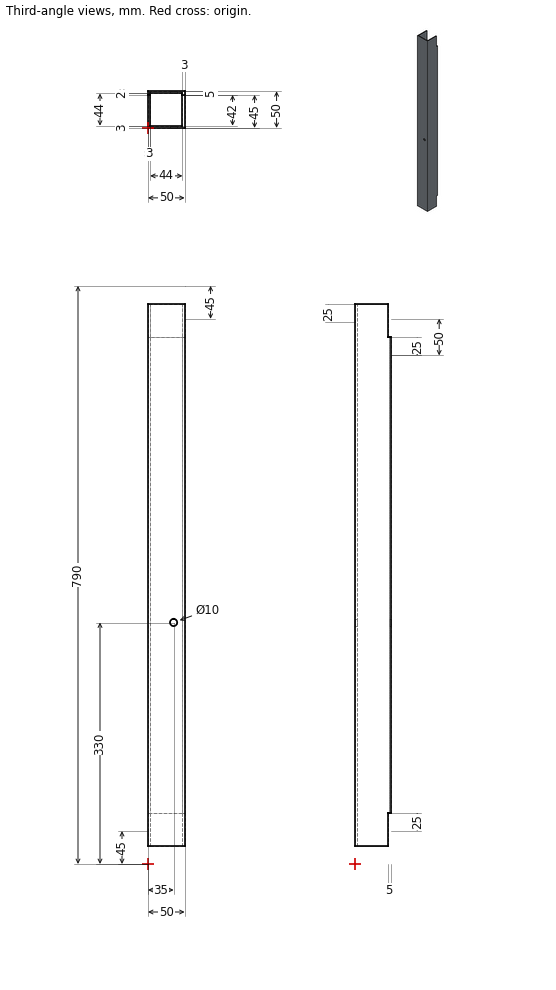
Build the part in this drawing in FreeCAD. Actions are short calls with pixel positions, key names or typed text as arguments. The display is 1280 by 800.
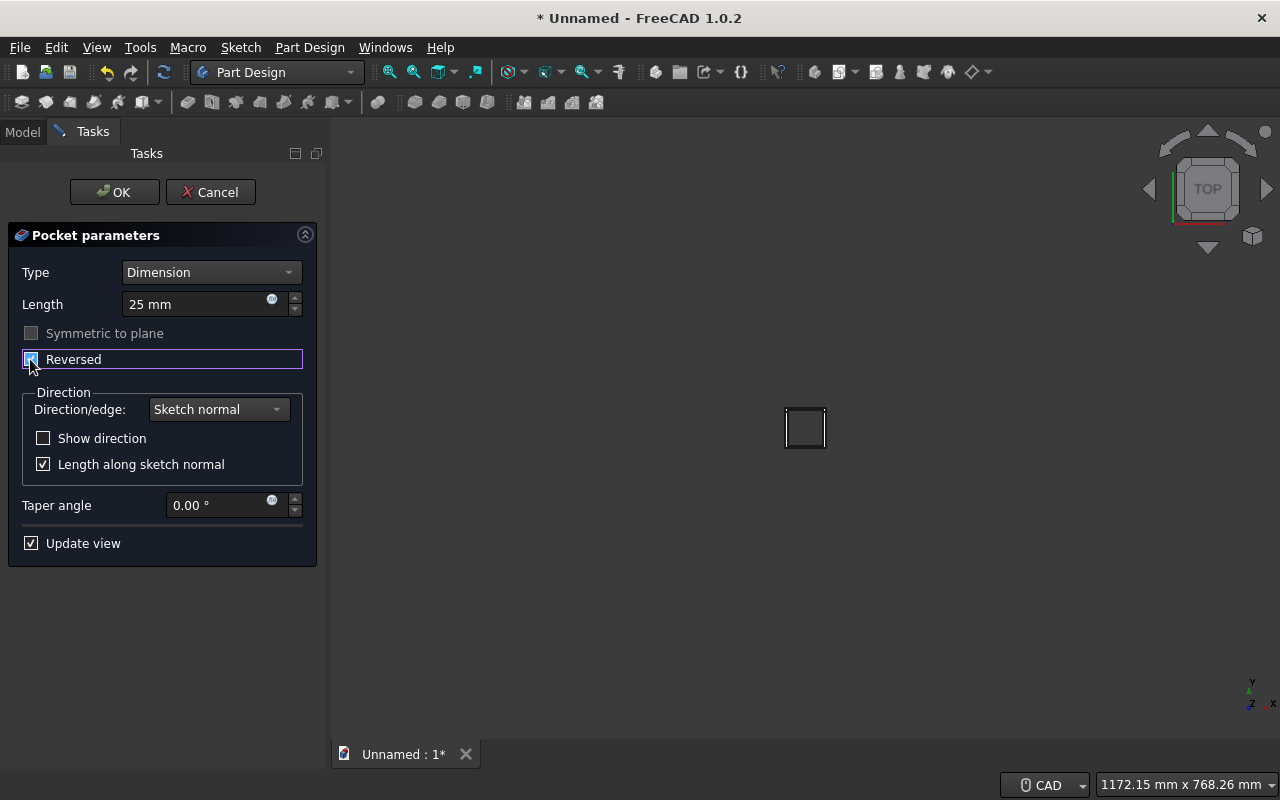
click(115, 192)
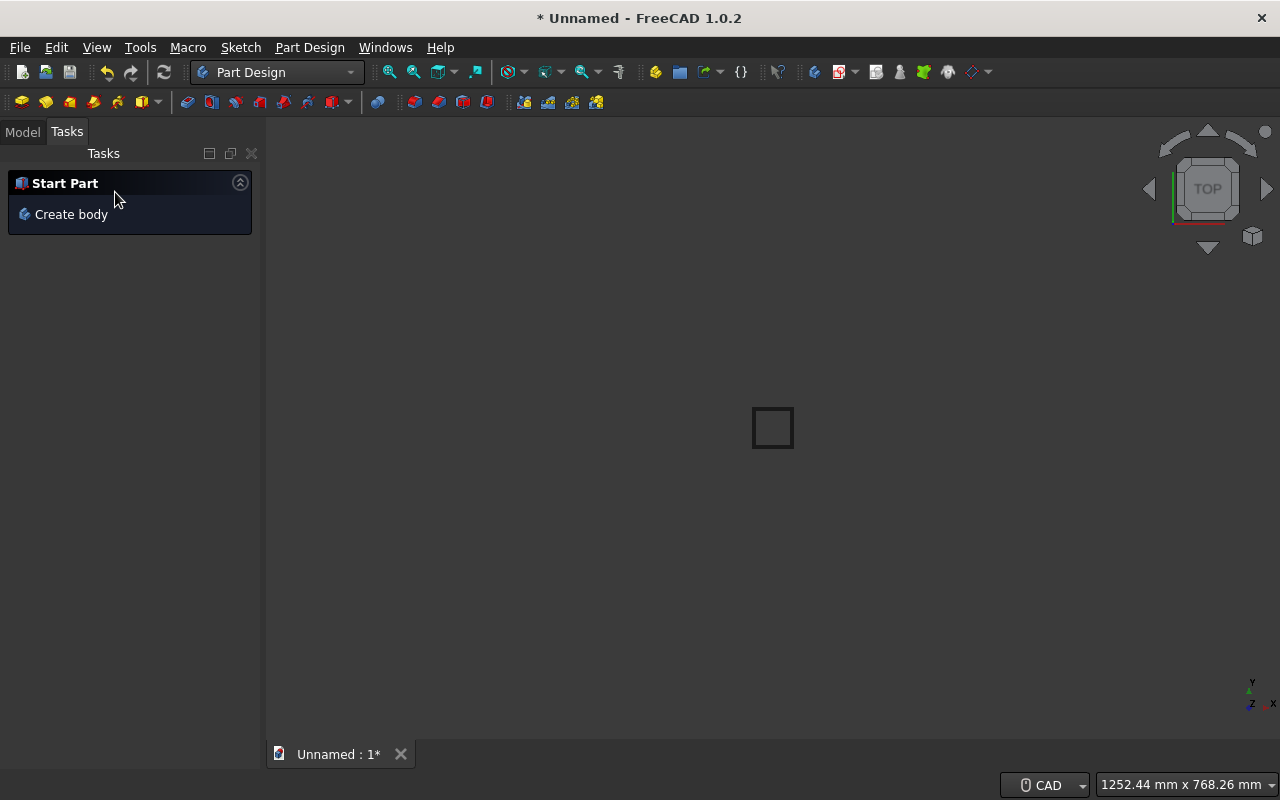
key(v)
key(f)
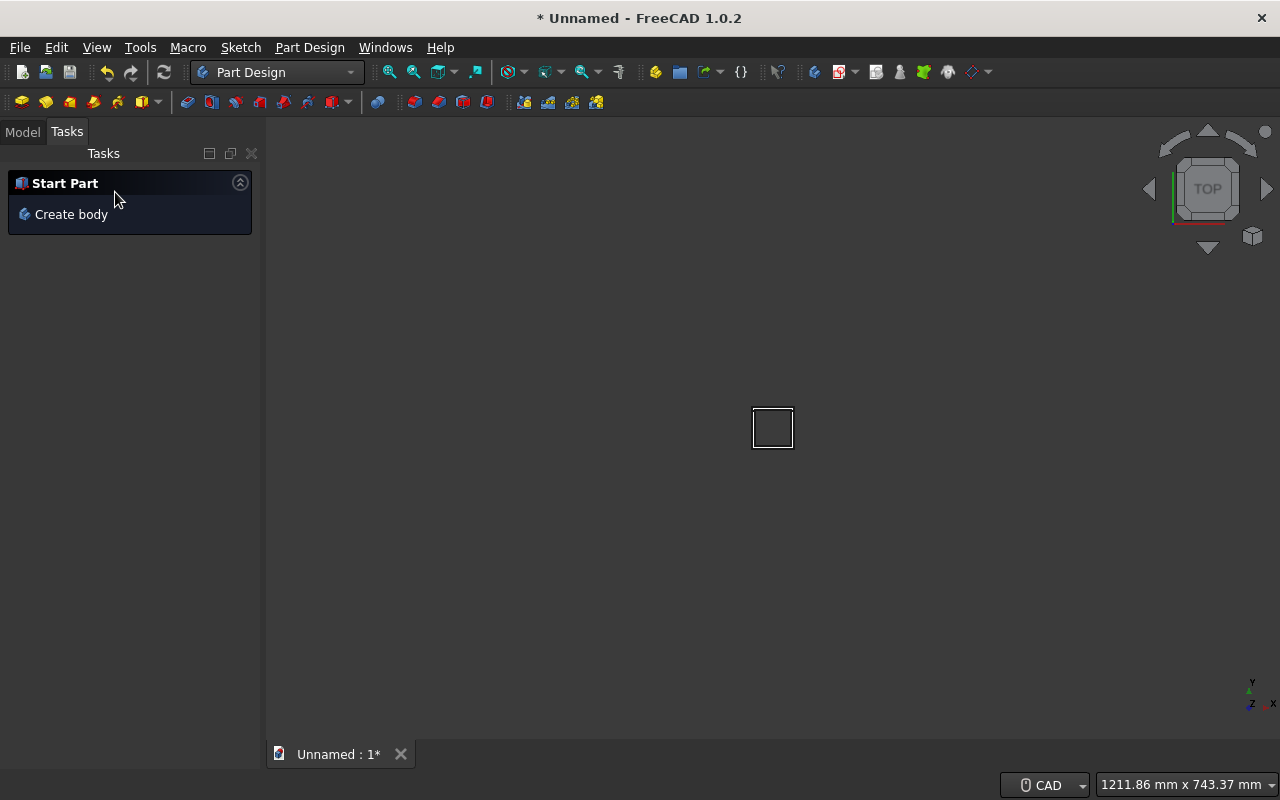
key(5)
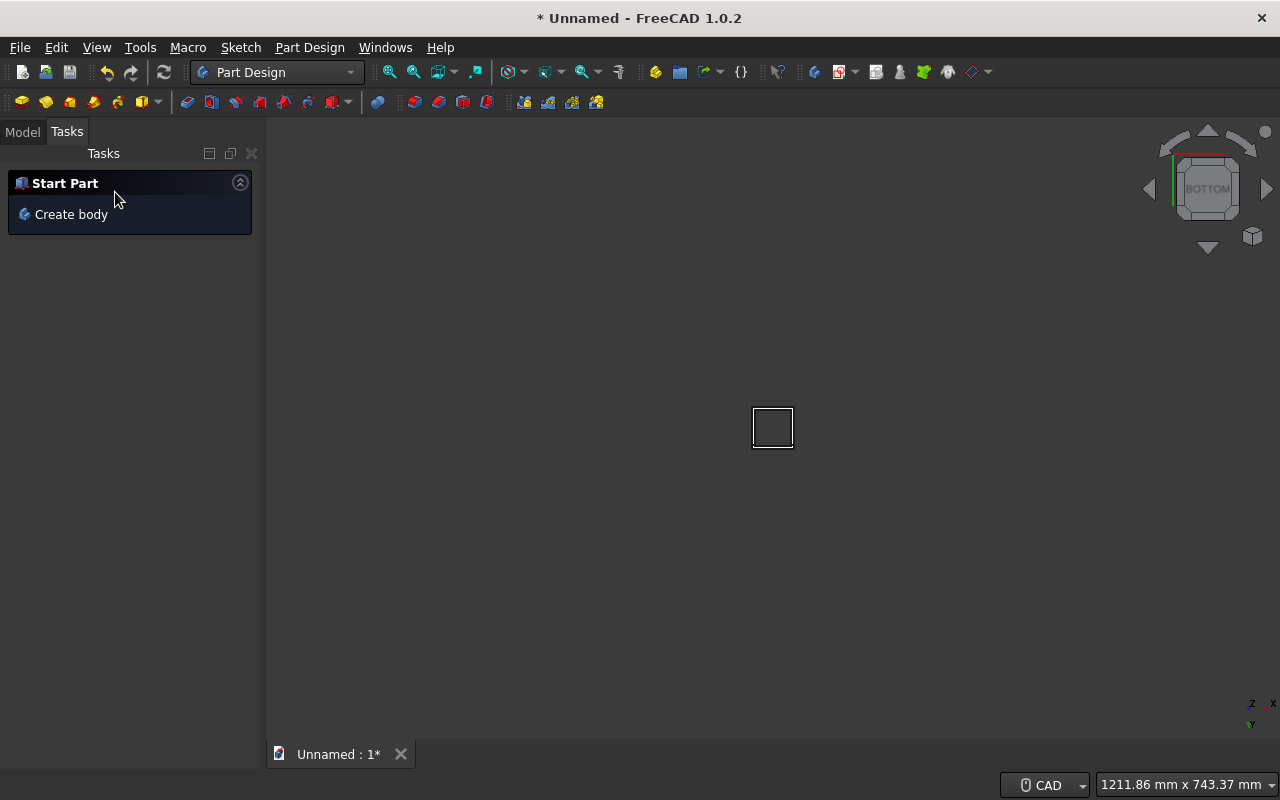
key(v)
key(f)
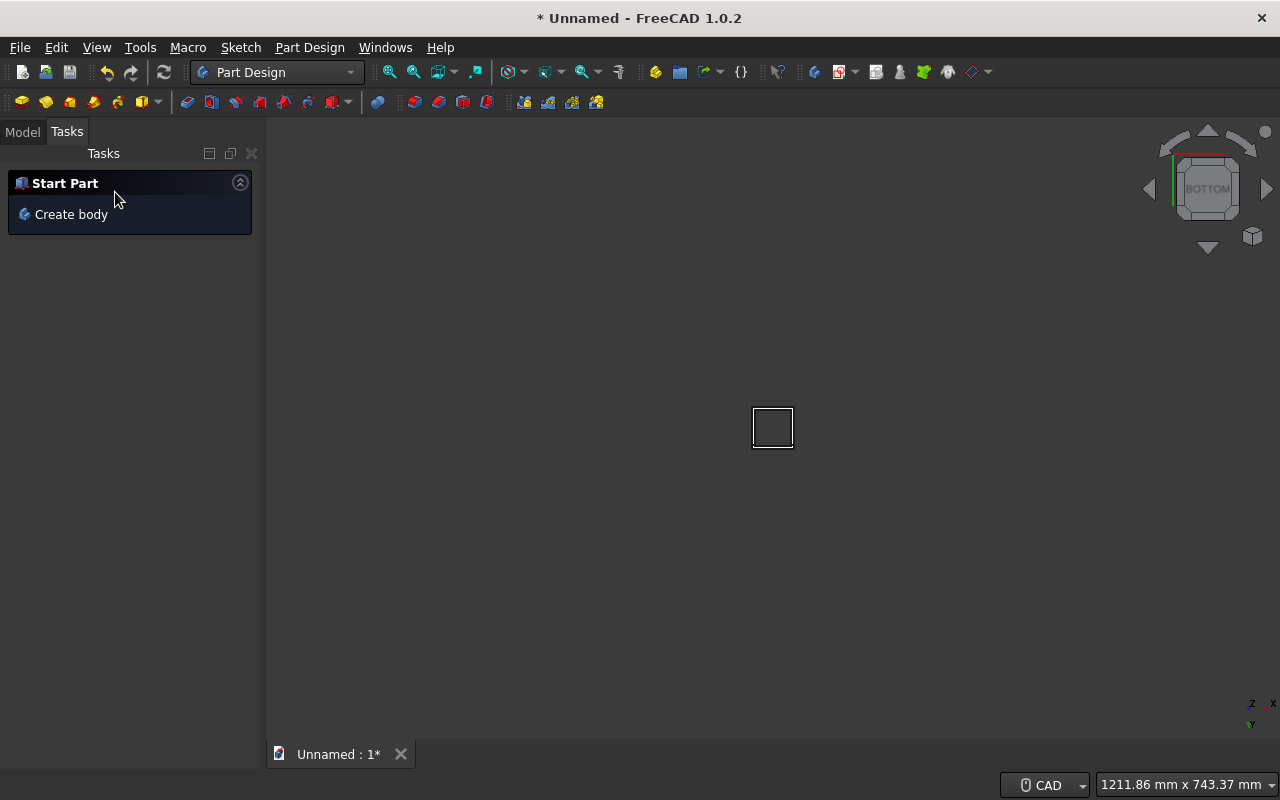
scroll(791, 446, up, 13)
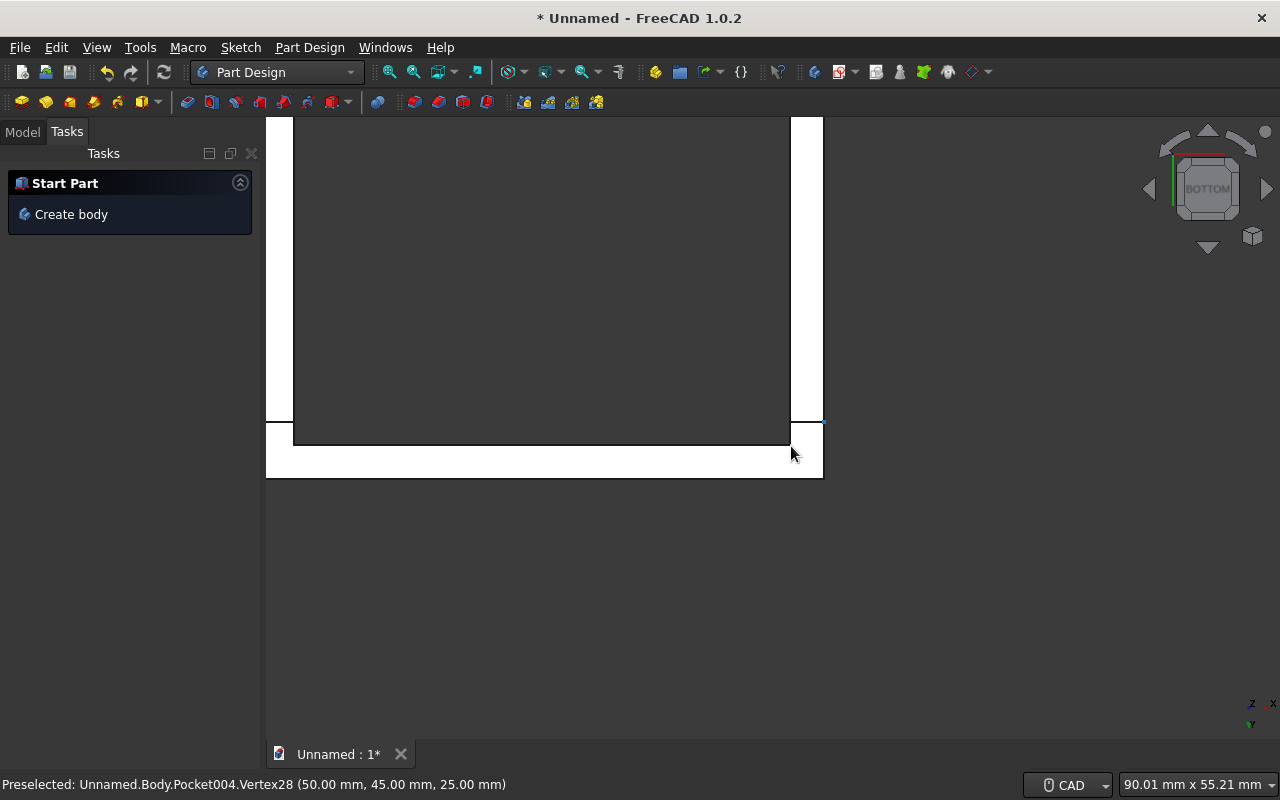
click(784, 458)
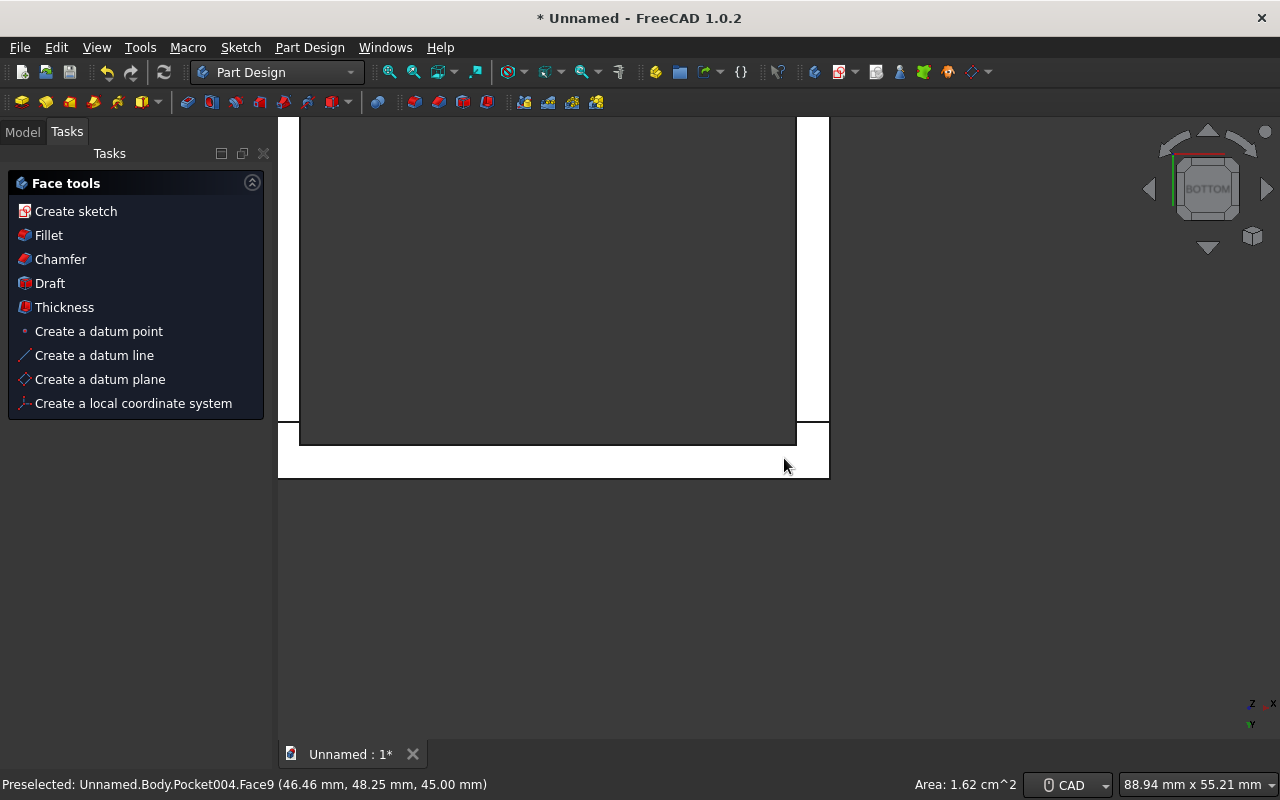
click(840, 72)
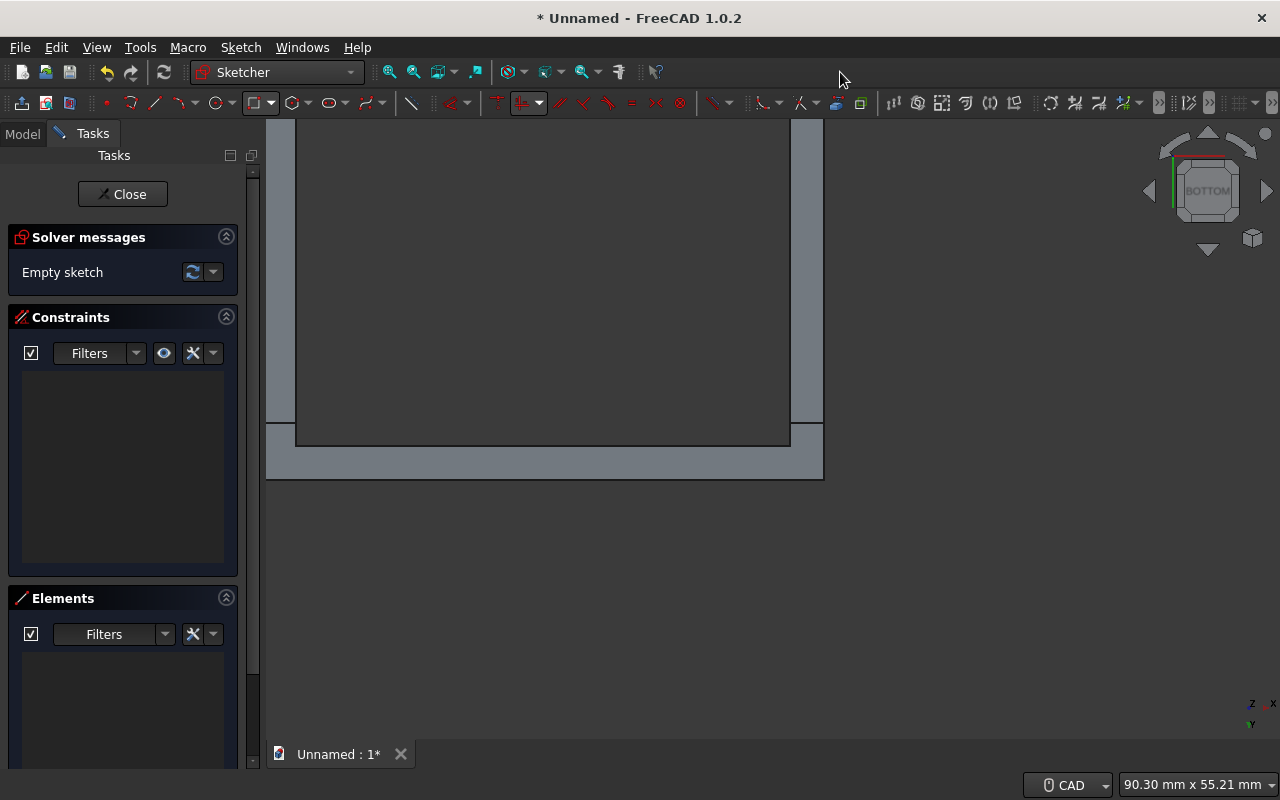
scroll(1033, 711, down, 2)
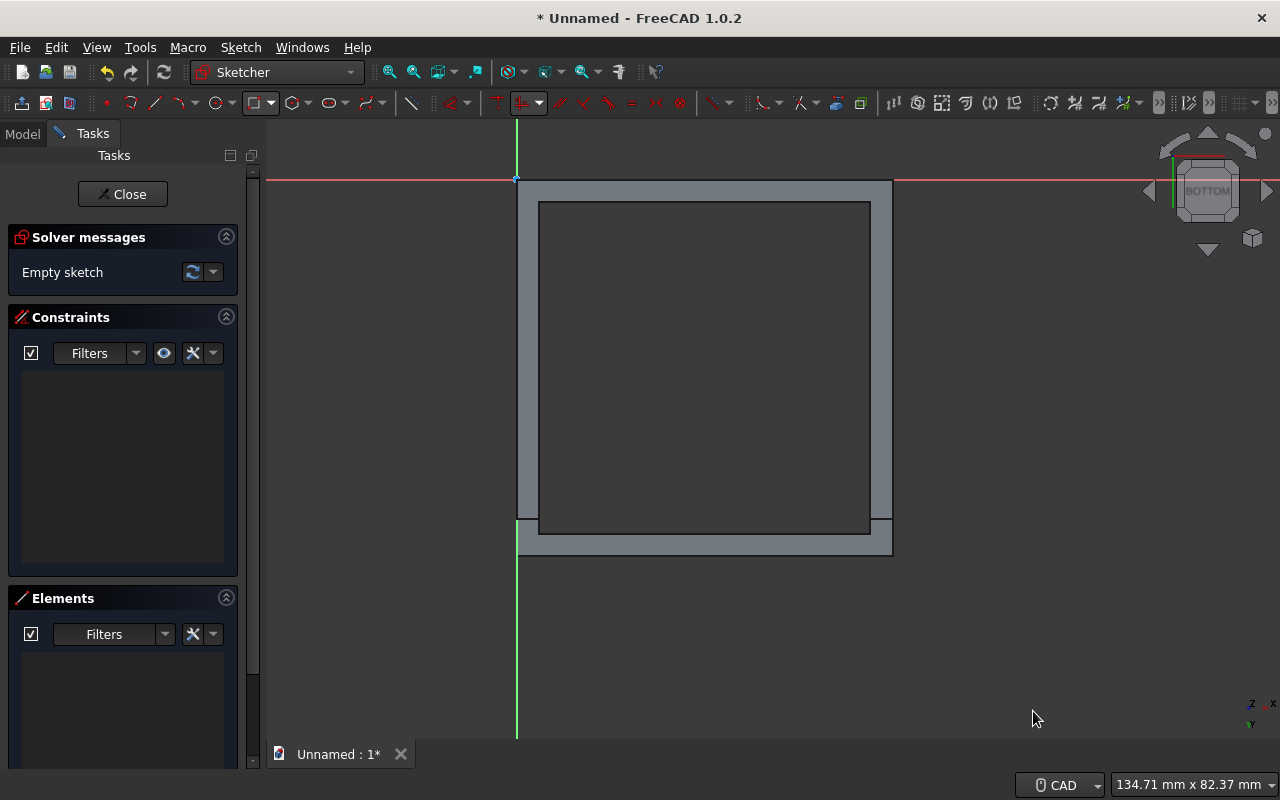
click(132, 104)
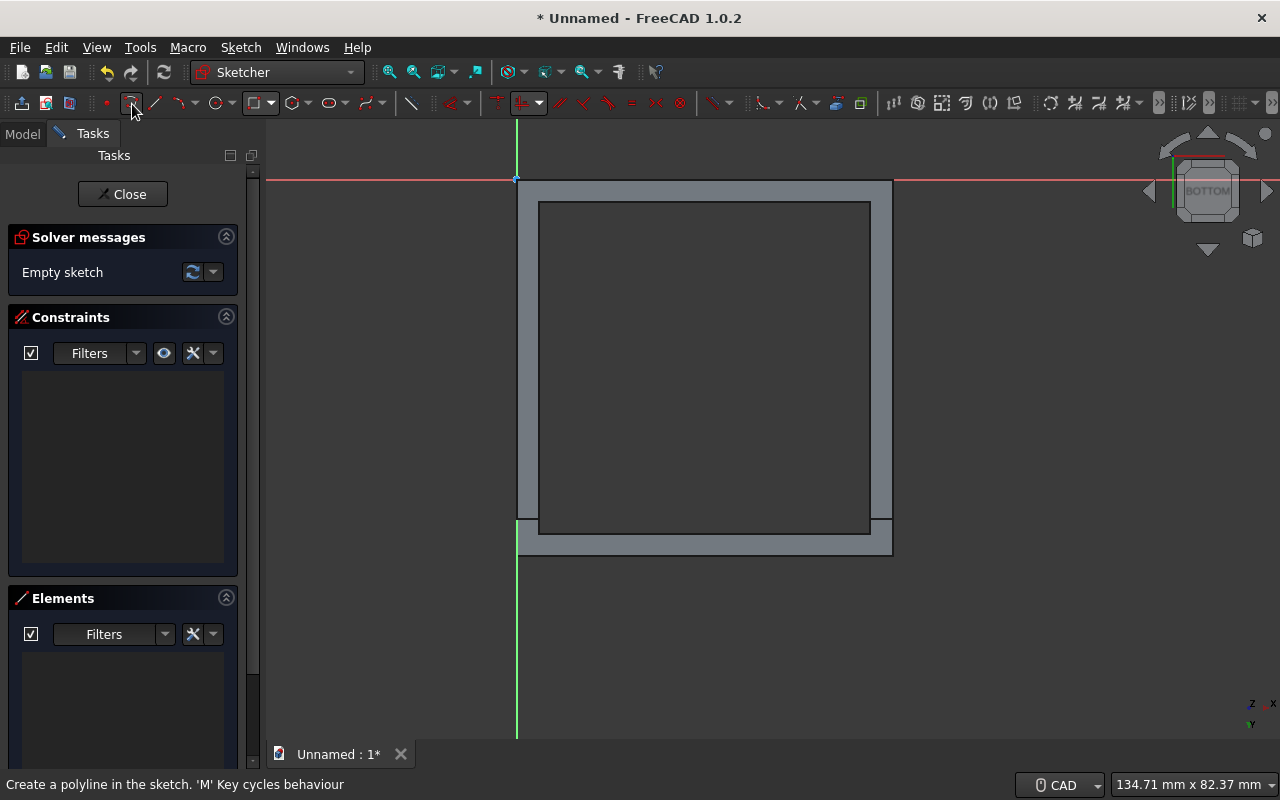
click(517, 519)
click(526, 556)
click(893, 556)
click(893, 519)
click(870, 519)
click(870, 534)
click(539, 534)
click(539, 519)
click(517, 520)
key(Escape)
key(Escape)